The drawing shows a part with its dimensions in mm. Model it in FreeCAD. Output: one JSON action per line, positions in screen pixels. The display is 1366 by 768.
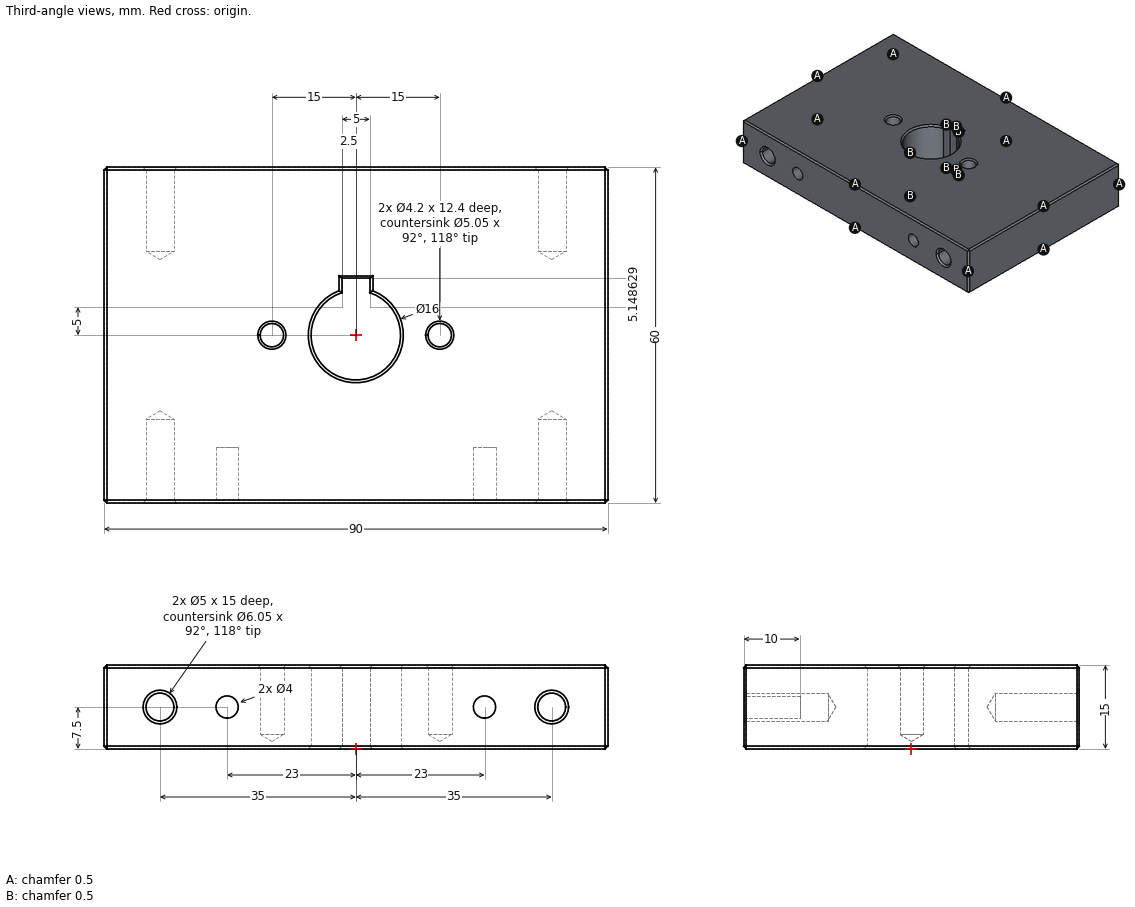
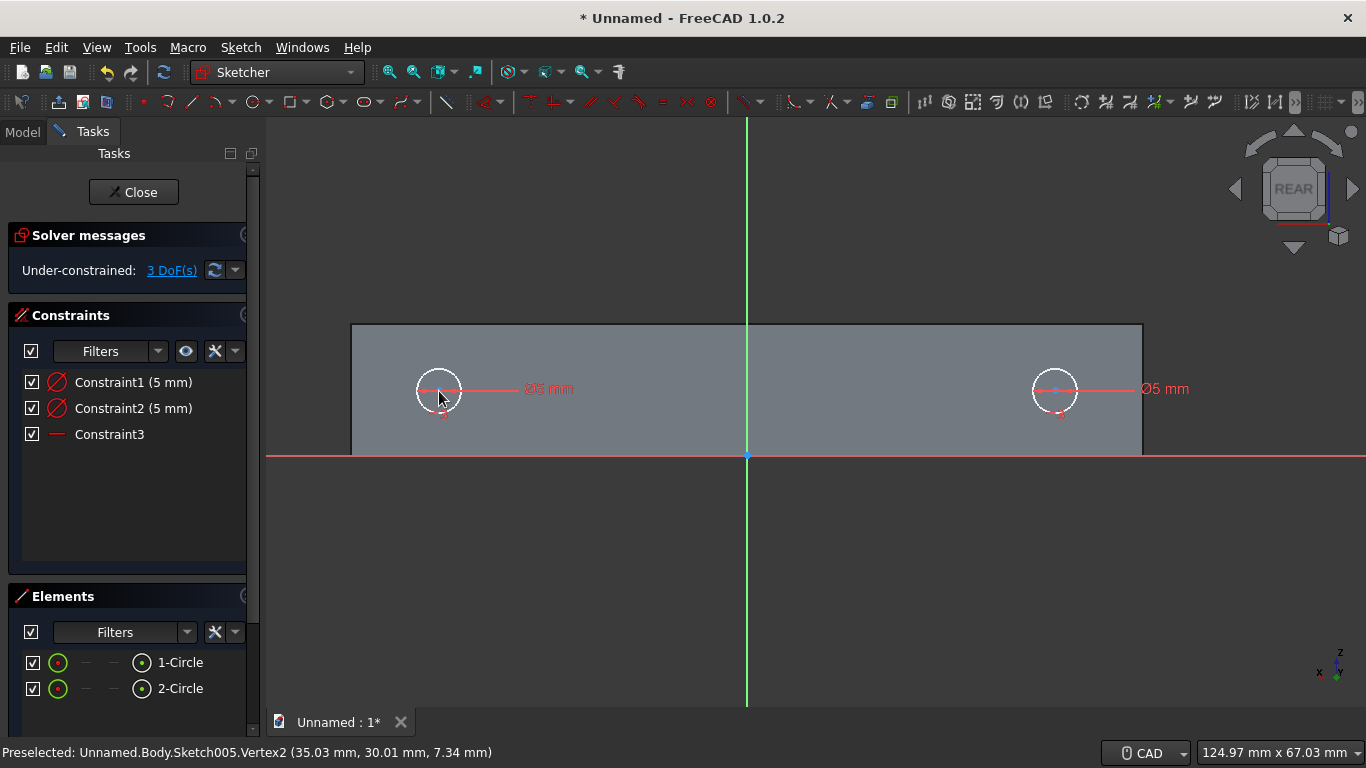
{"action": "left_click", "coordinate": [484, 102]}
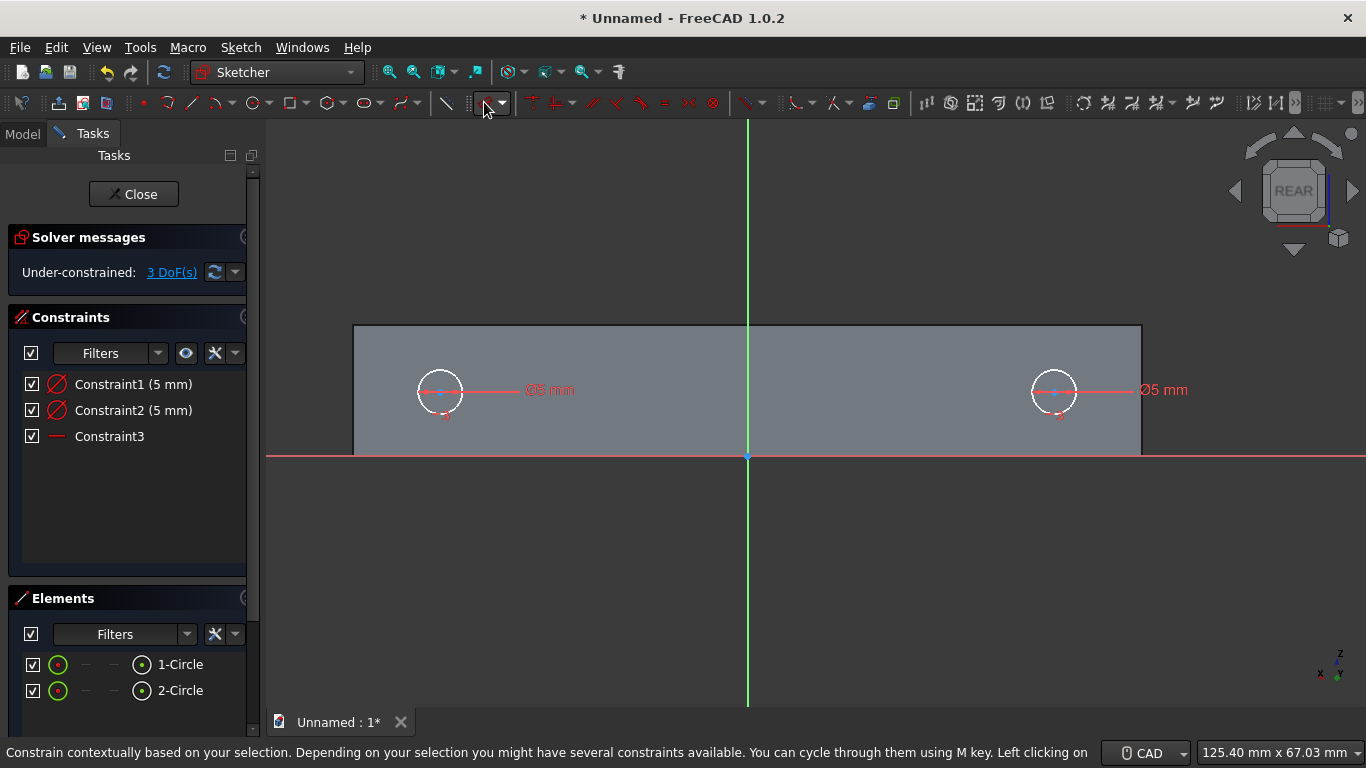
{"action": "left_click", "coordinate": [1054, 392]}
{"action": "left_click", "coordinate": [901, 490]}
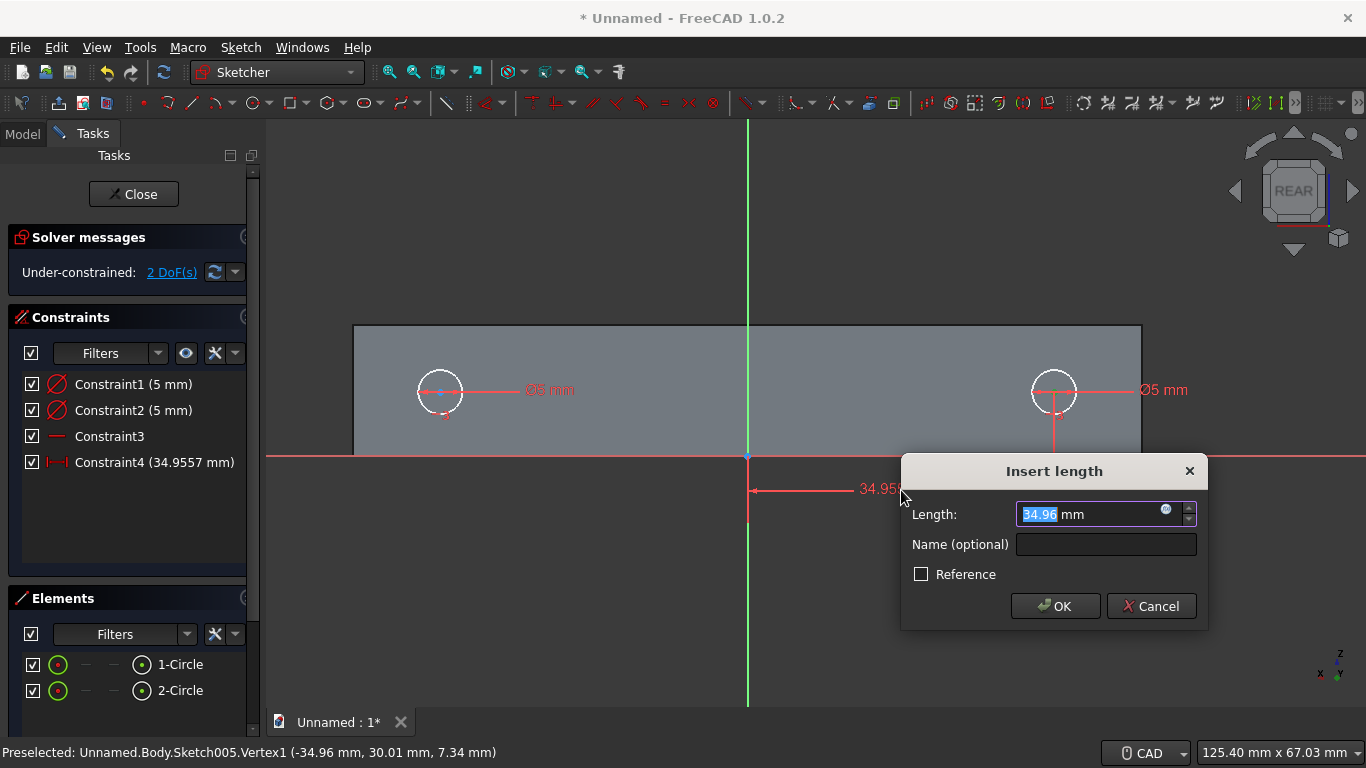
{"action": "type", "text": "35"}
{"action": "key", "text": "Return"}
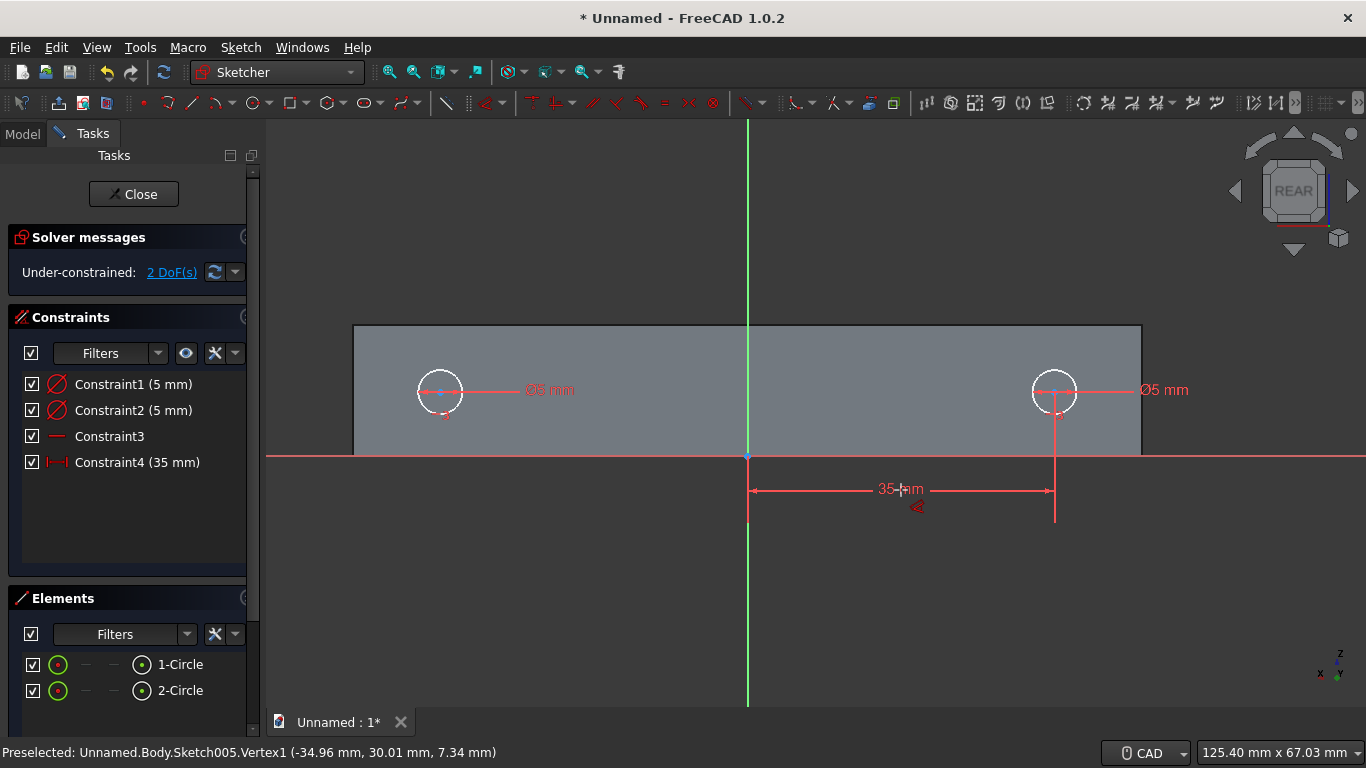
{"action": "left_click", "coordinate": [440, 392]}
{"action": "left_click", "coordinate": [594, 490]}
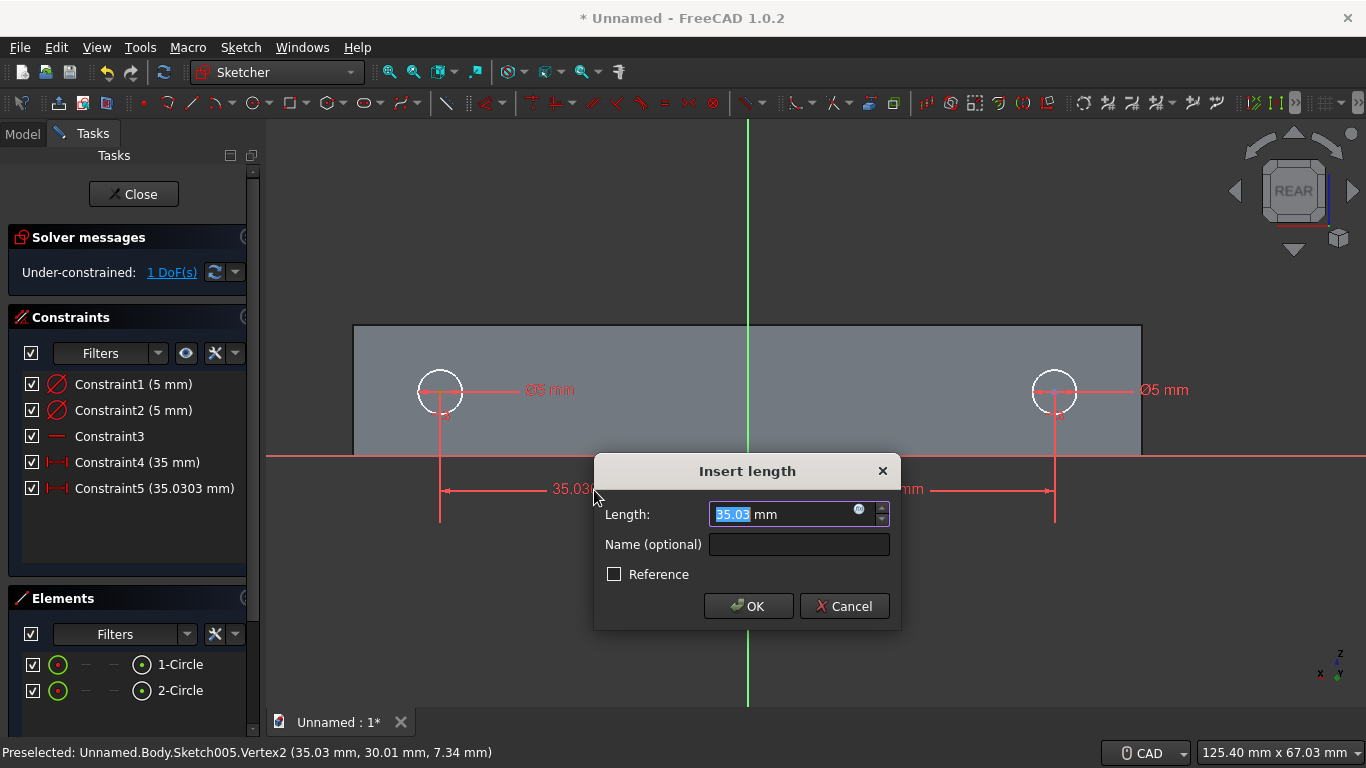
{"action": "type", "text": "35"}
{"action": "key", "text": "Return"}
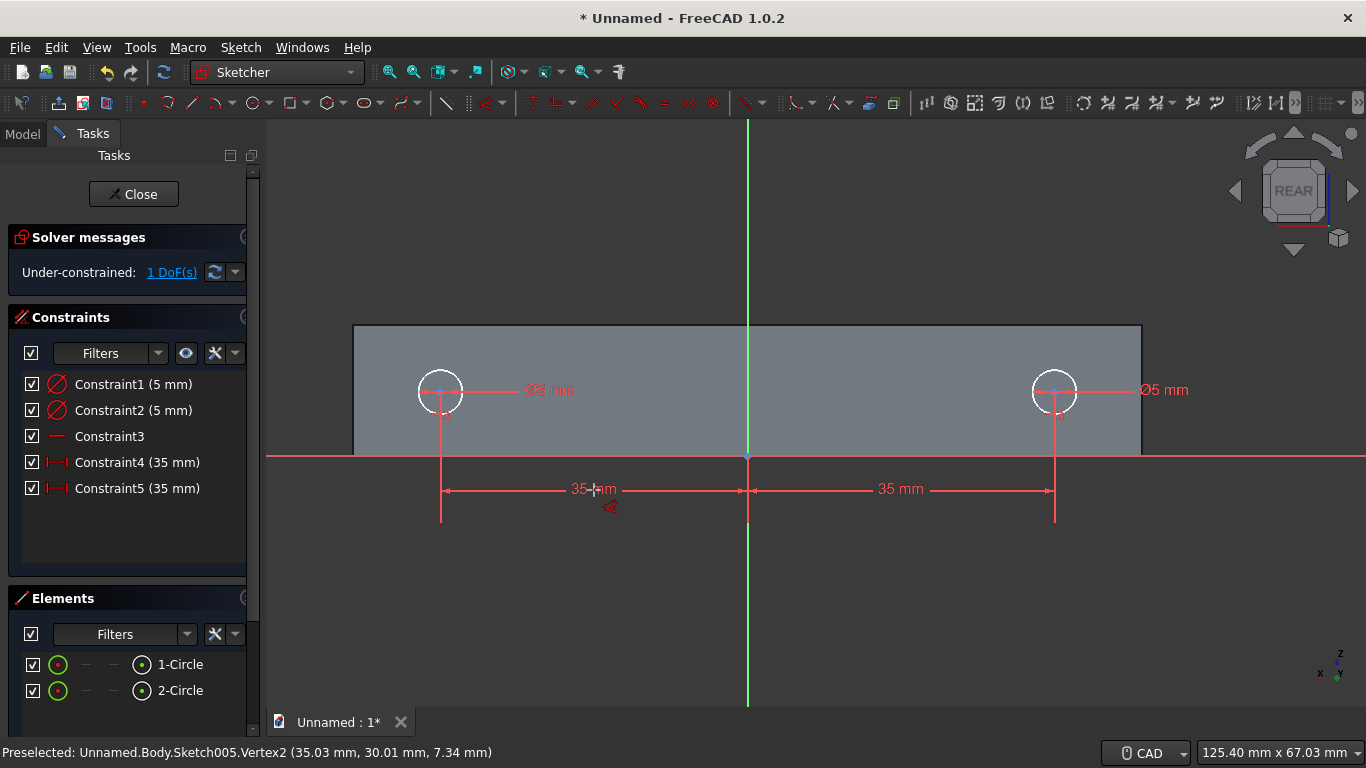
{"action": "left_click", "coordinate": [1055, 392]}
{"action": "left_click", "coordinate": [1089, 424]}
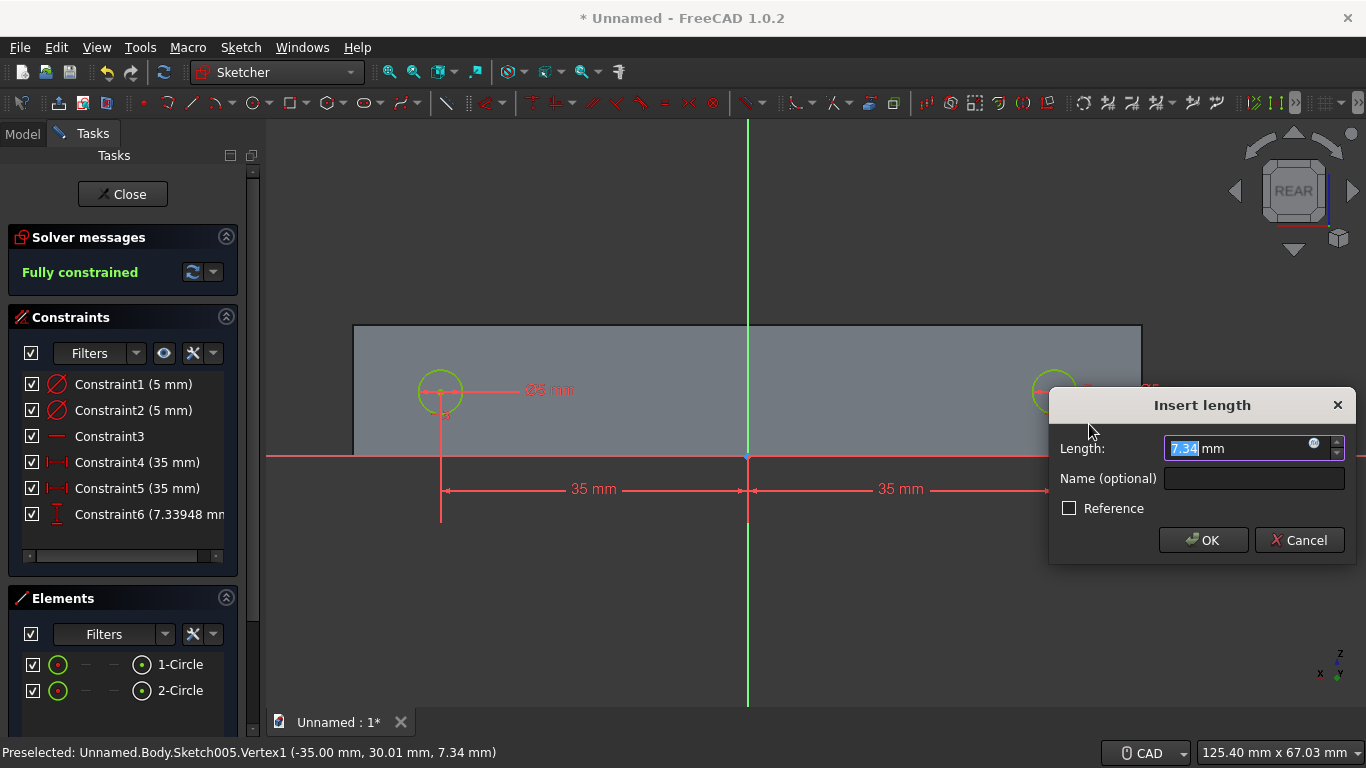
{"action": "type", "text": "7.5"}
{"action": "key", "text": "Return"}
{"action": "key", "text": "Escape"}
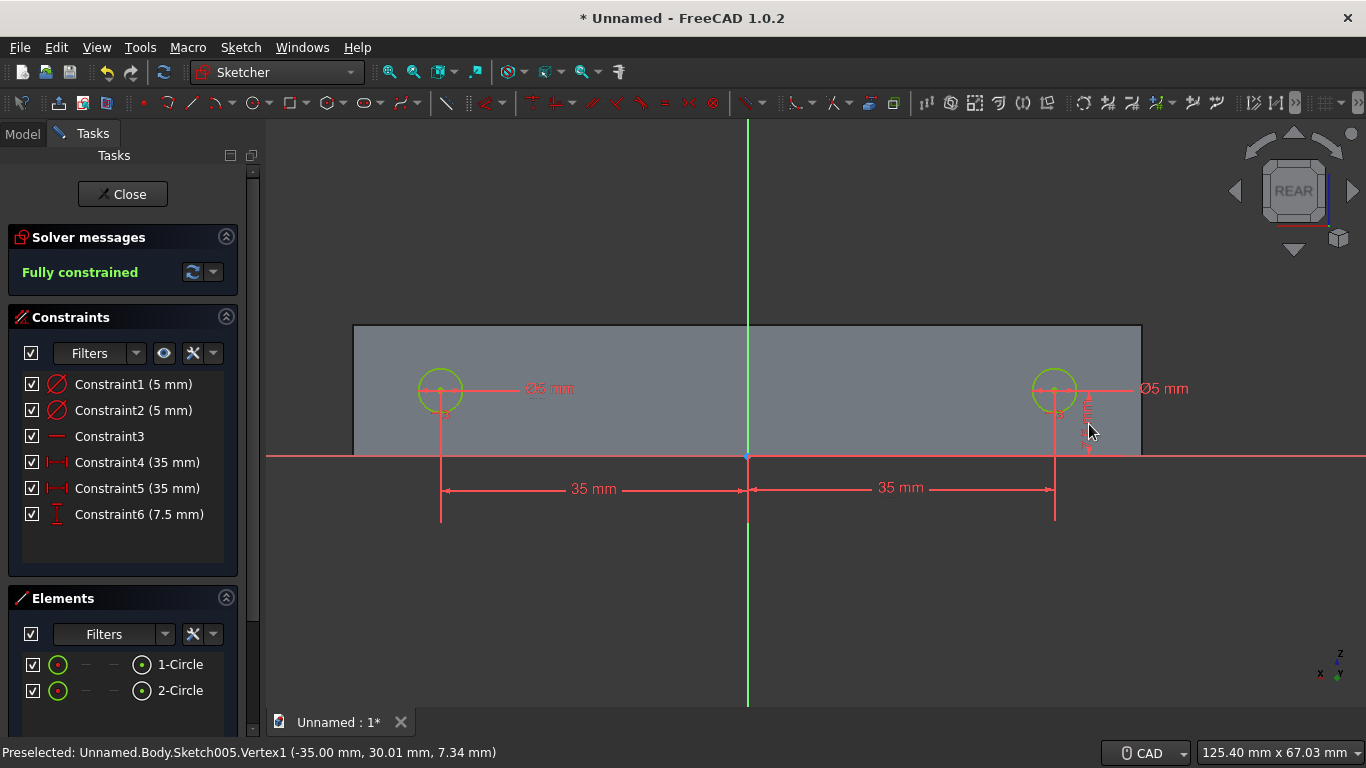
{"action": "left_click", "coordinate": [123, 194]}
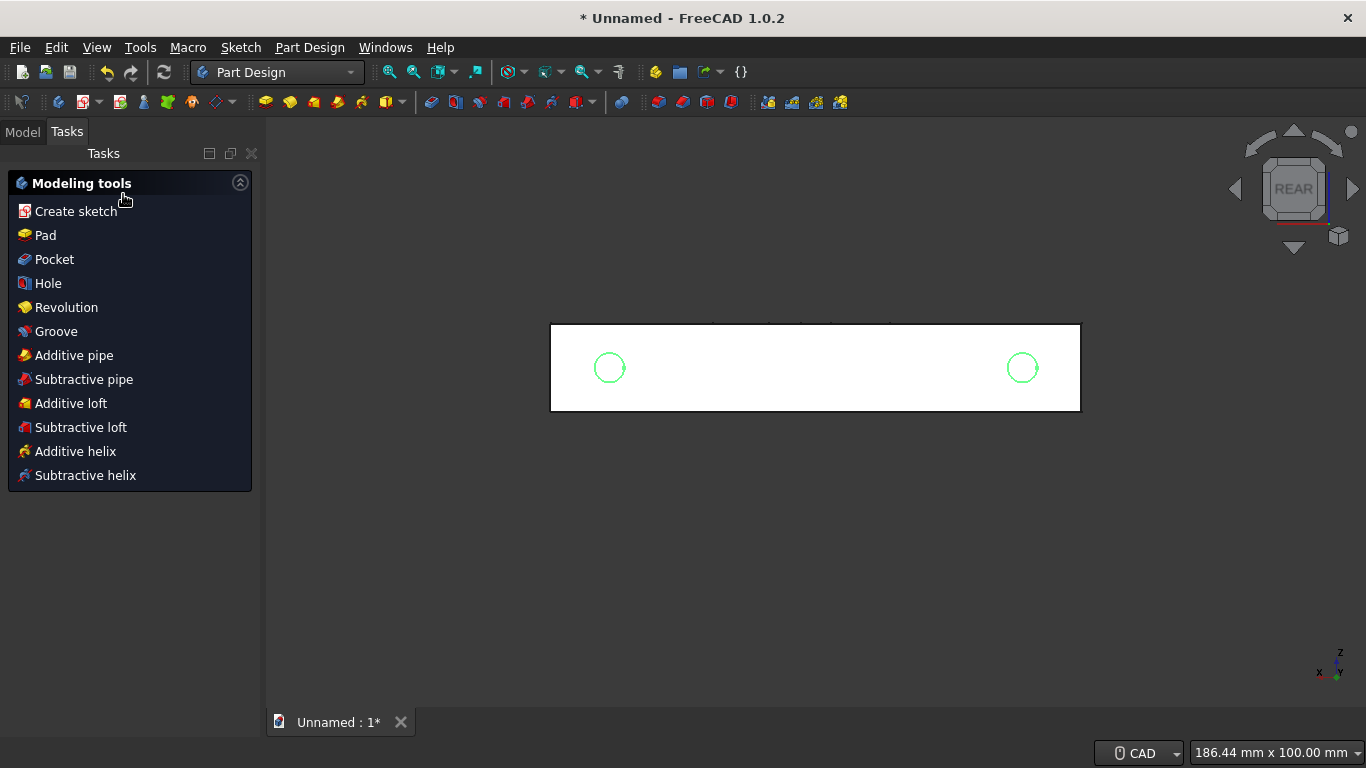
{"action": "left_click", "coordinate": [456, 102]}